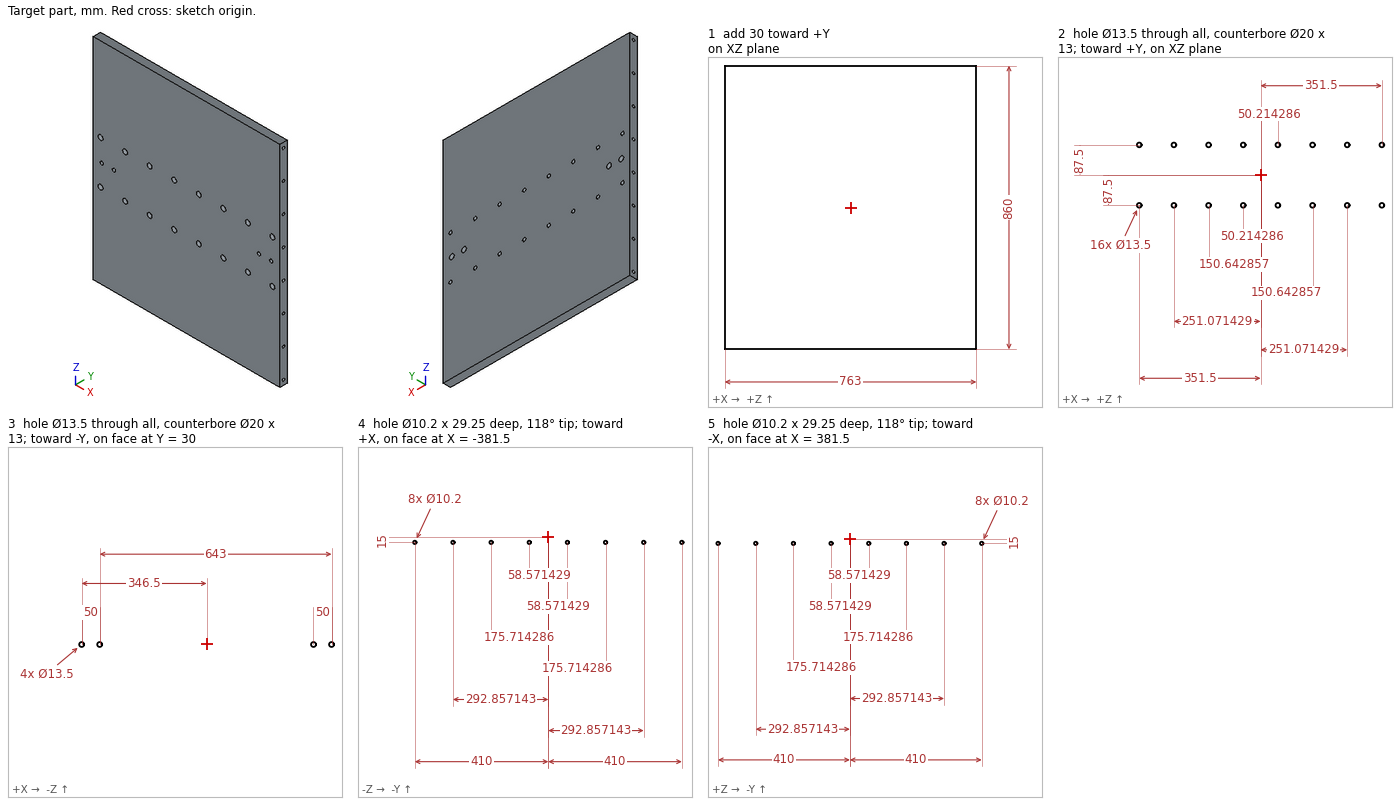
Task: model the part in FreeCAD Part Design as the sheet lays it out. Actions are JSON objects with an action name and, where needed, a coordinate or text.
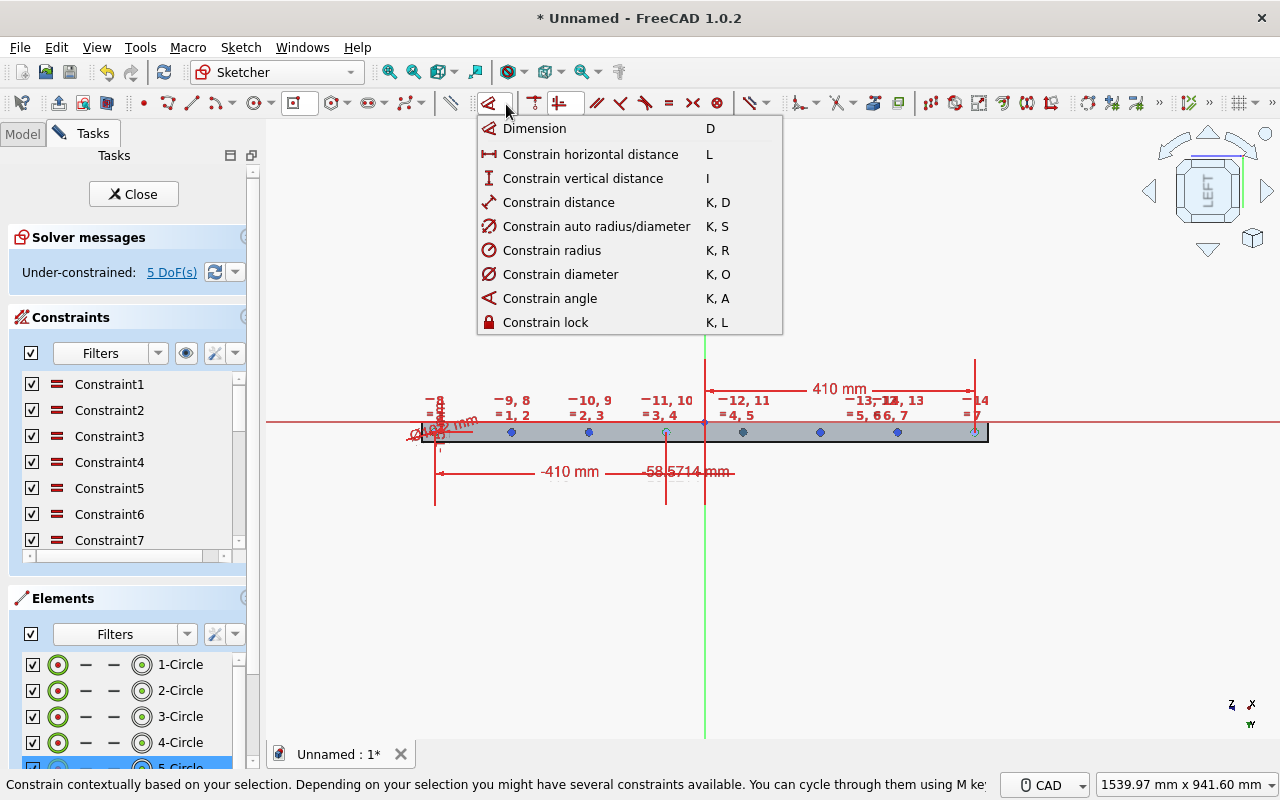
{"action": "left_click", "coordinate": [630, 154]}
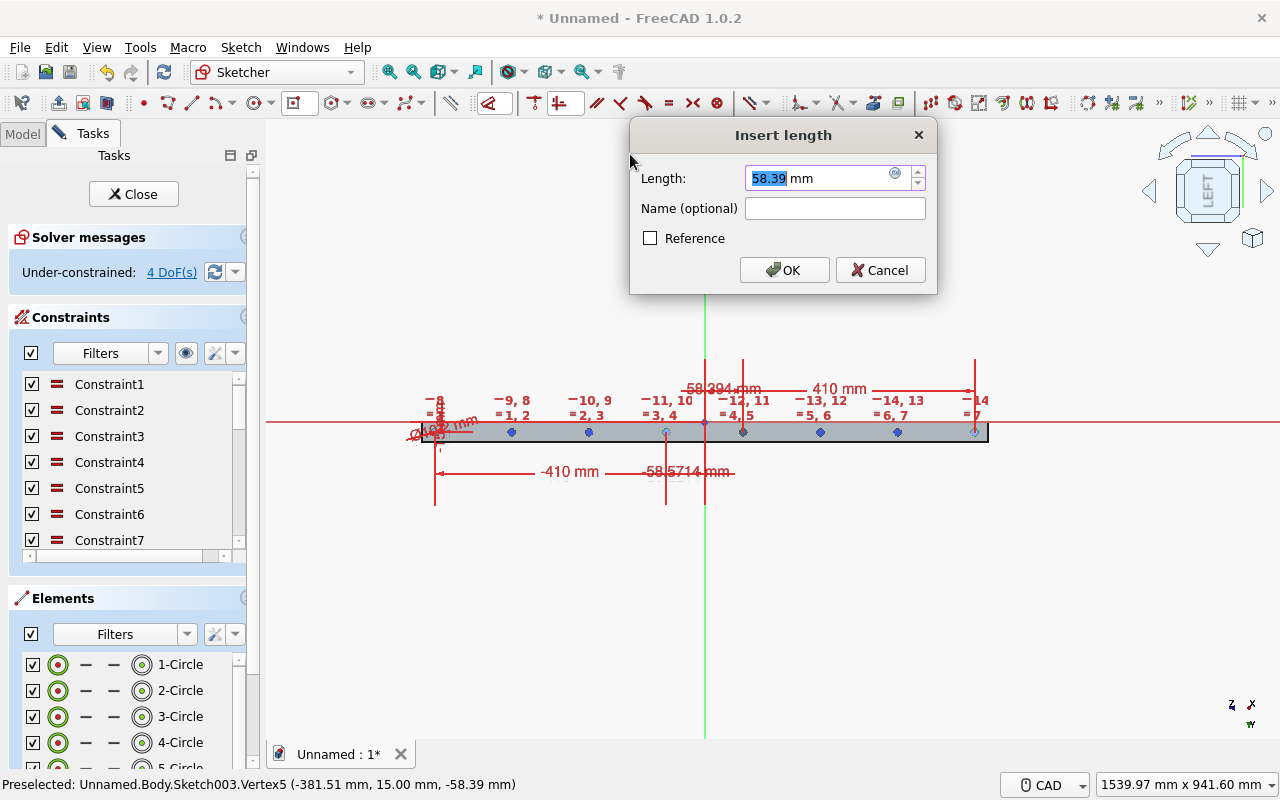
{"action": "type", "text": "58.571429"}
{"action": "key", "text": "Return"}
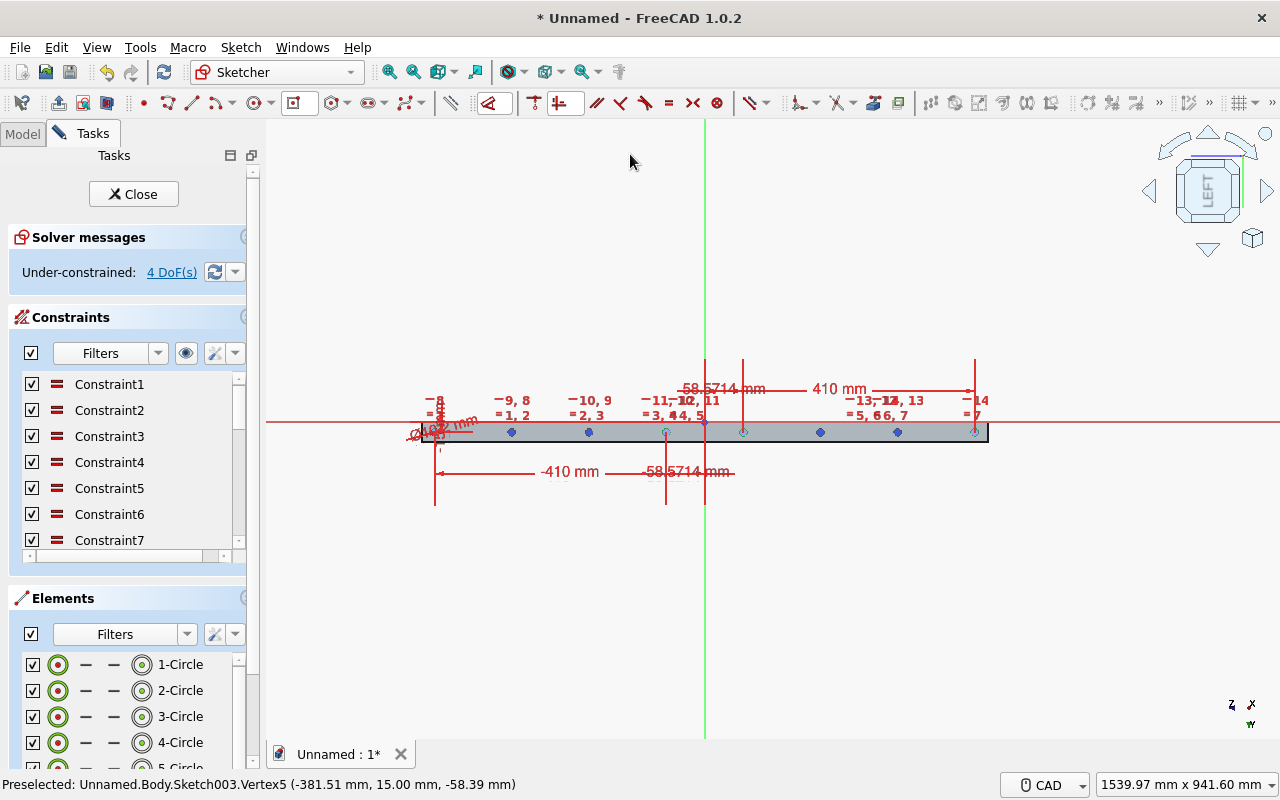
{"action": "left_click", "coordinate": [512, 432]}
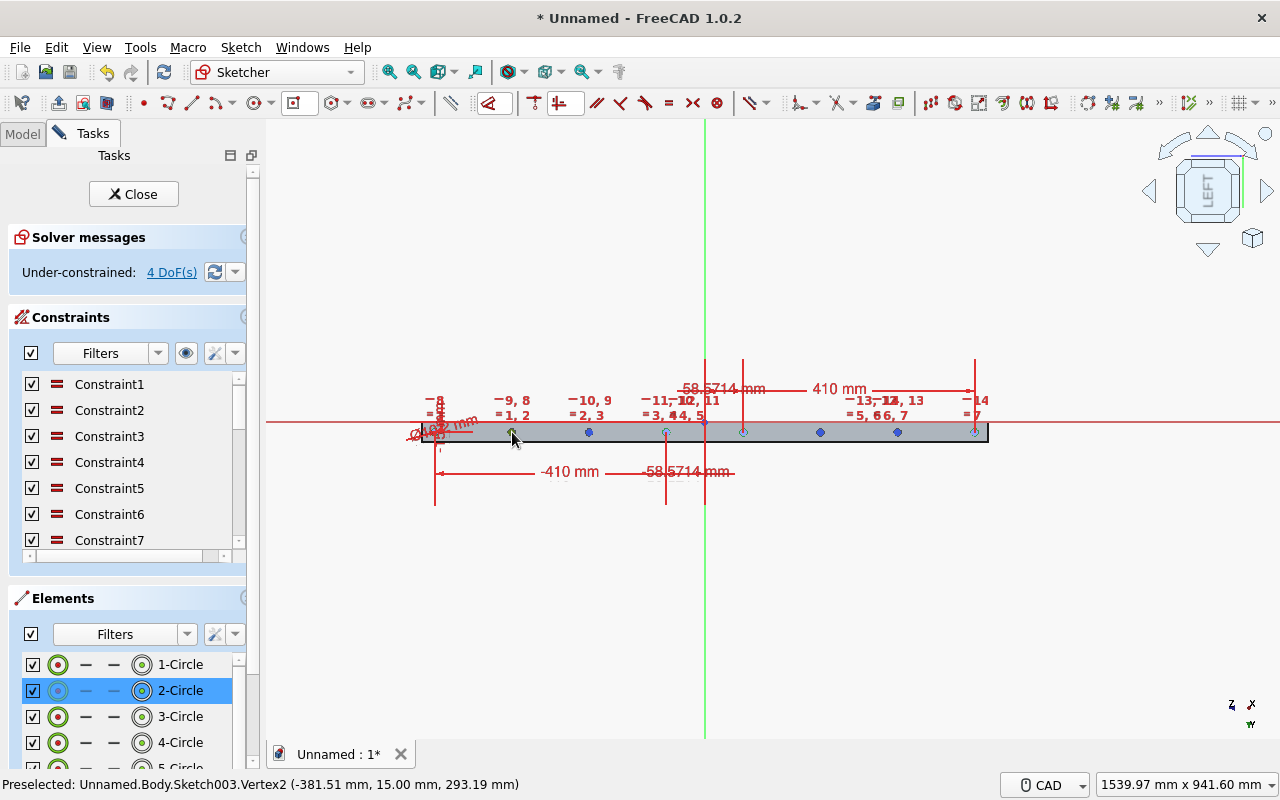
{"action": "key", "text": "l"}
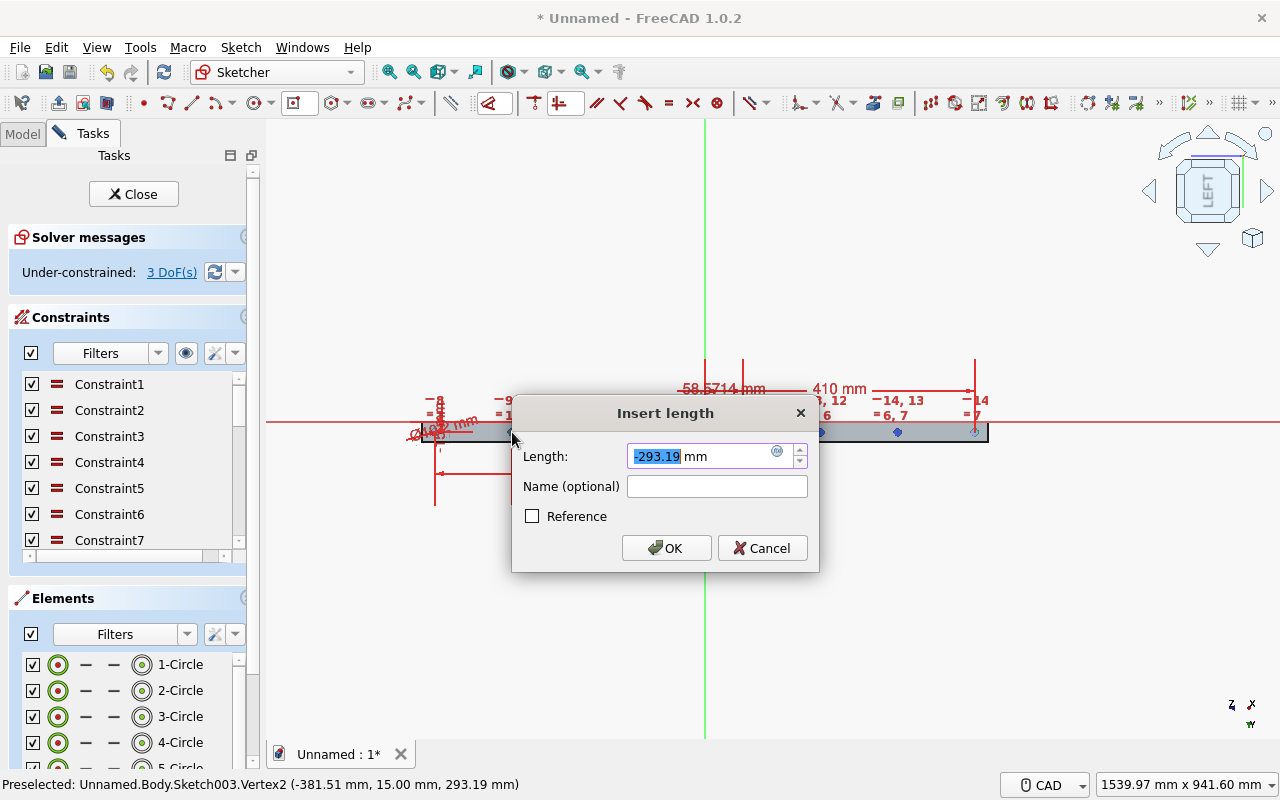
{"action": "type", "text": "-292.857143"}
{"action": "key", "text": "Return"}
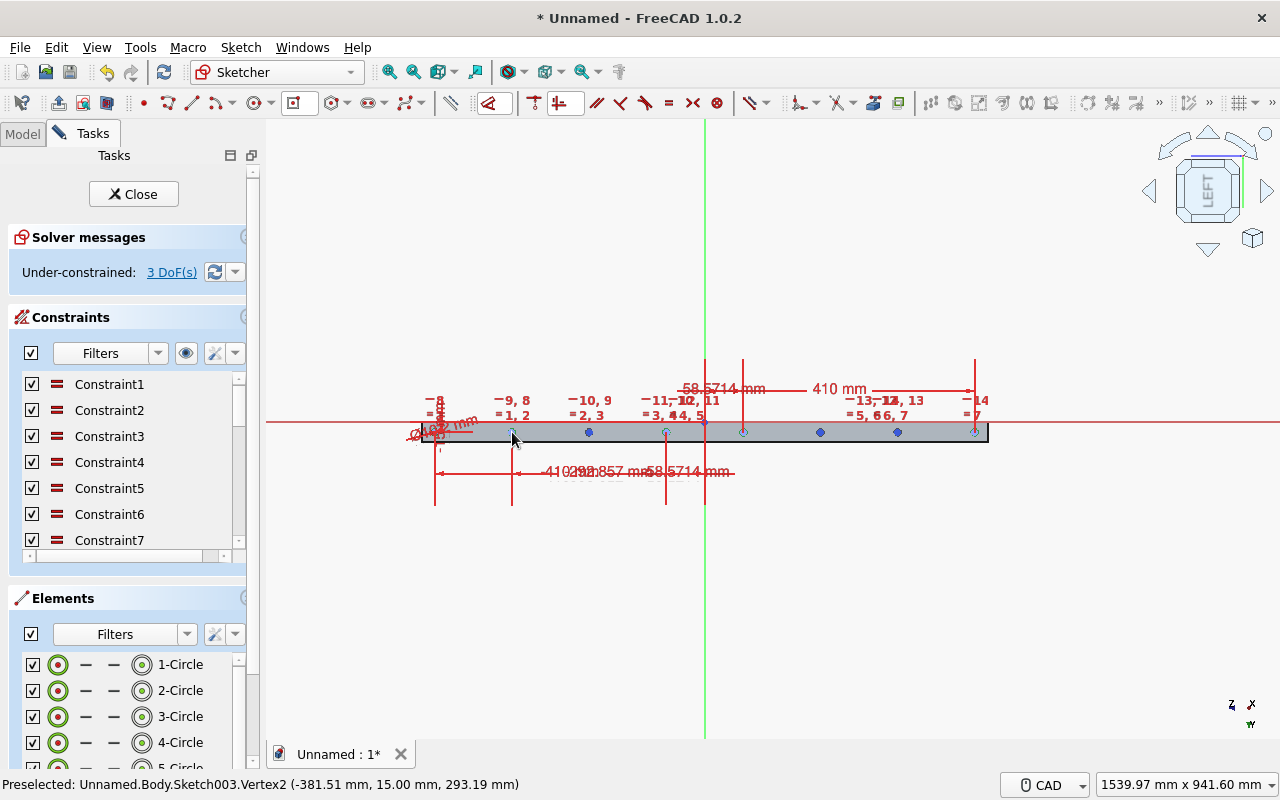
{"action": "left_click", "coordinate": [589, 432]}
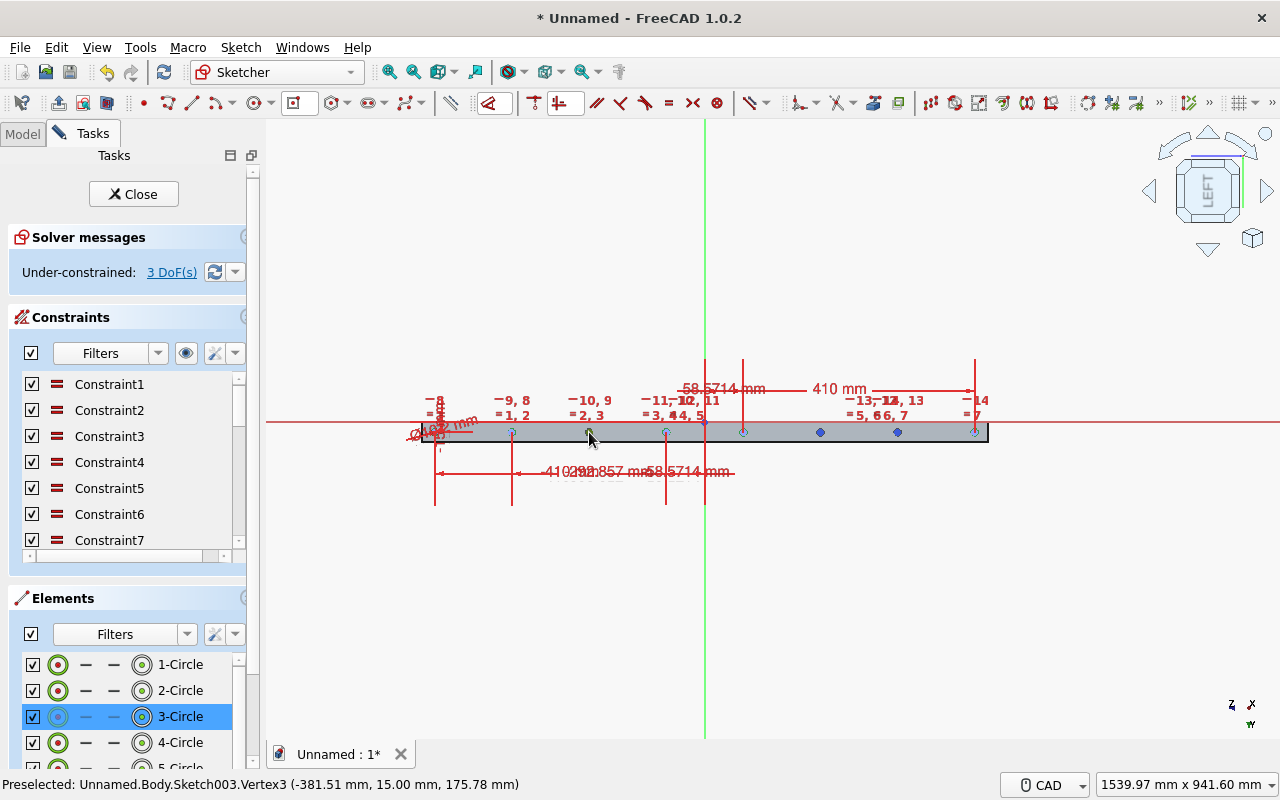
{"action": "left_click", "coordinate": [506, 104]}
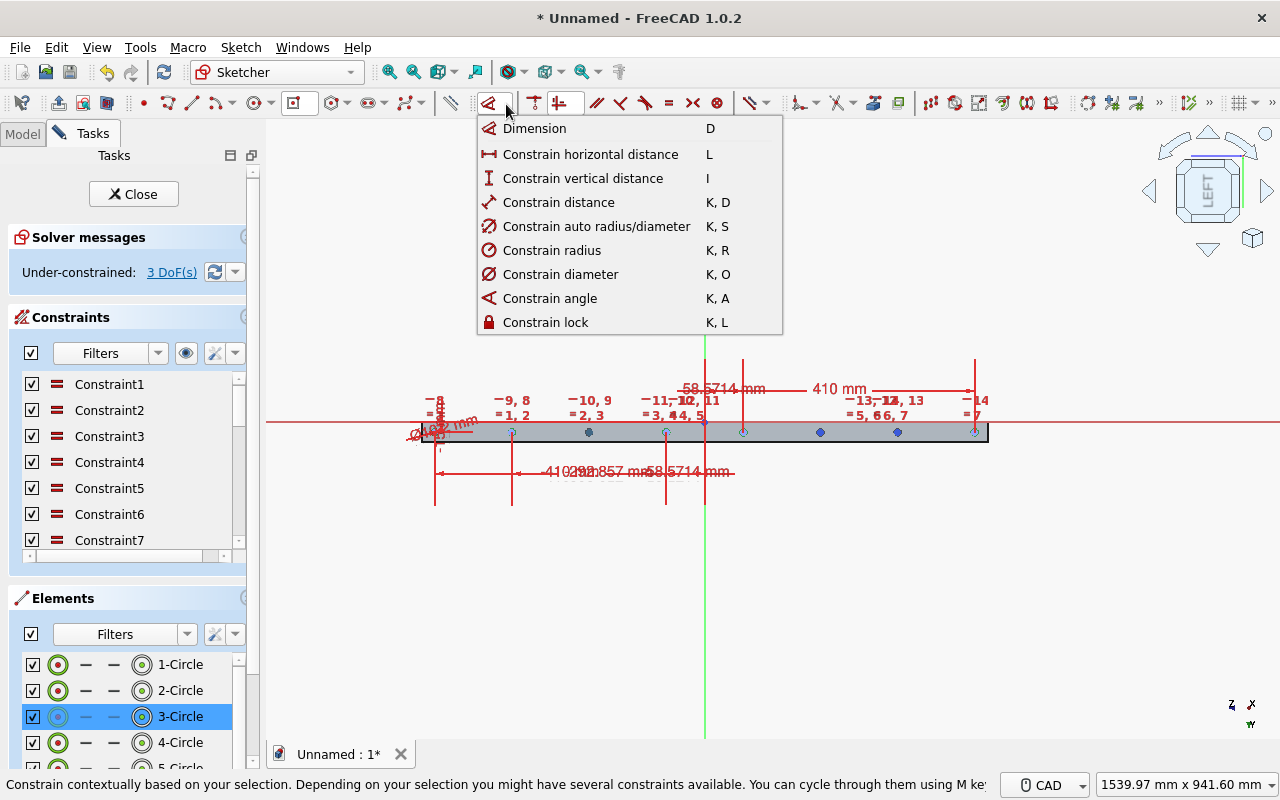
{"action": "left_click", "coordinate": [630, 154]}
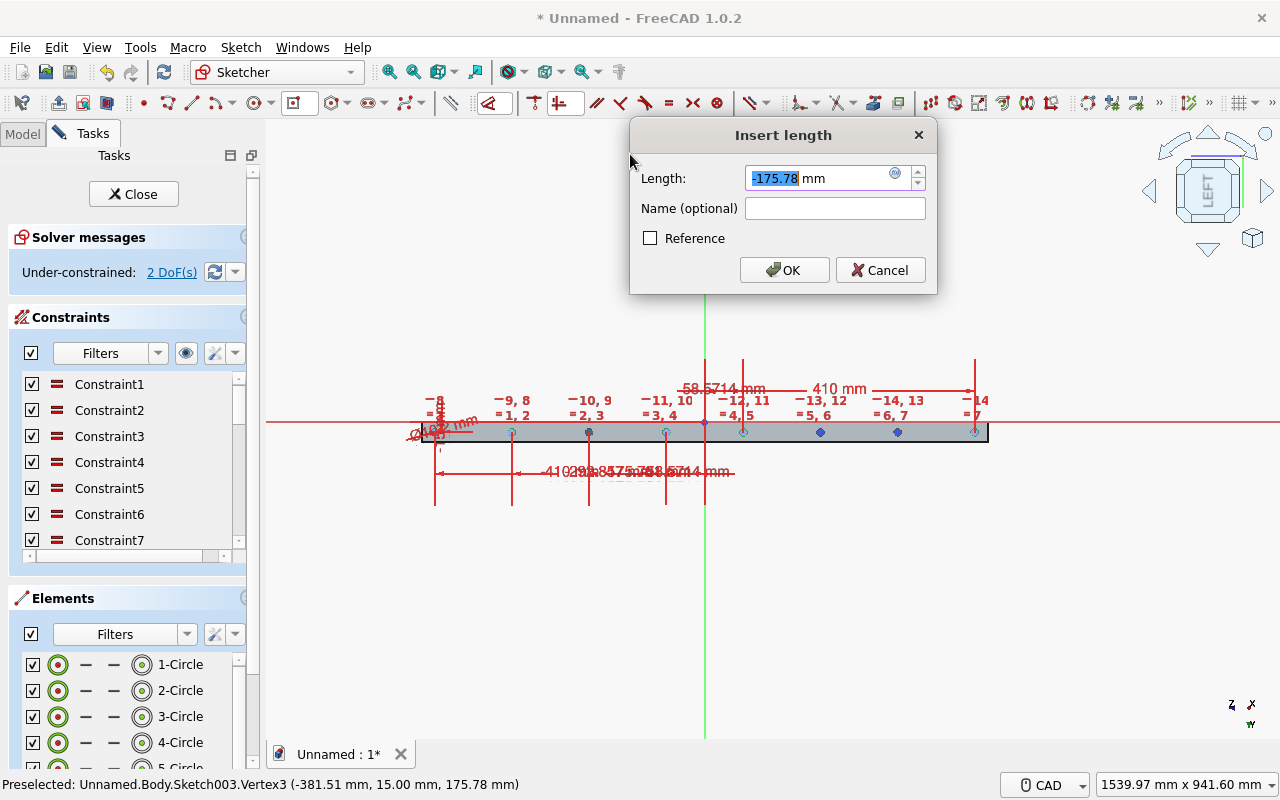
{"action": "type", "text": "-175.714286"}
{"action": "key", "text": "Return"}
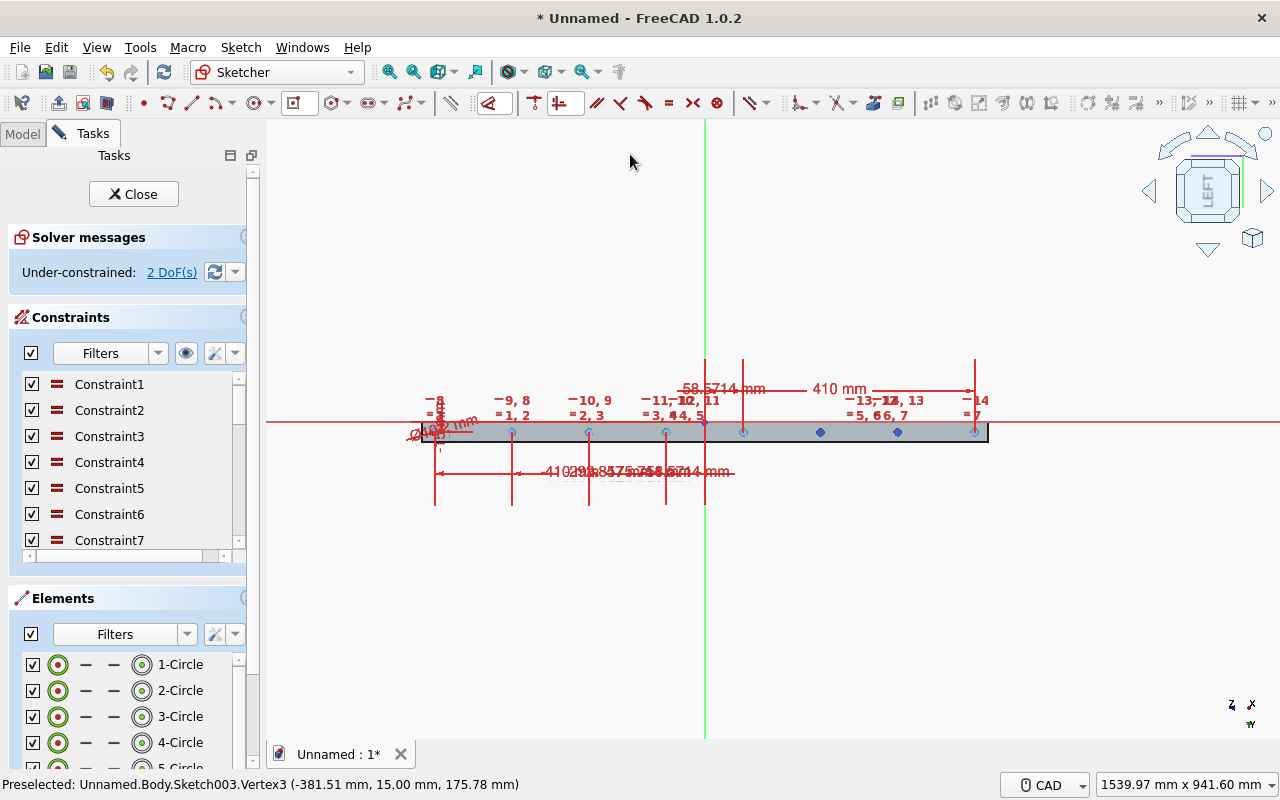
{"action": "left_click", "coordinate": [820, 432]}